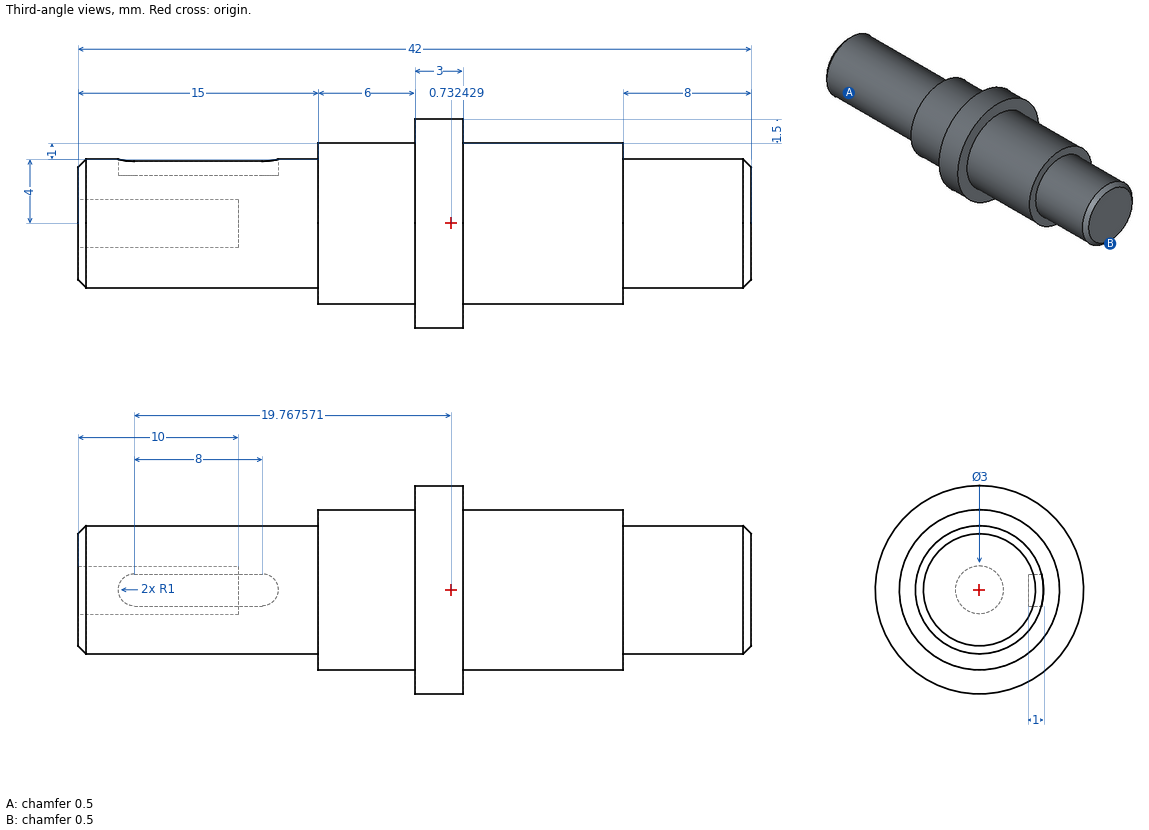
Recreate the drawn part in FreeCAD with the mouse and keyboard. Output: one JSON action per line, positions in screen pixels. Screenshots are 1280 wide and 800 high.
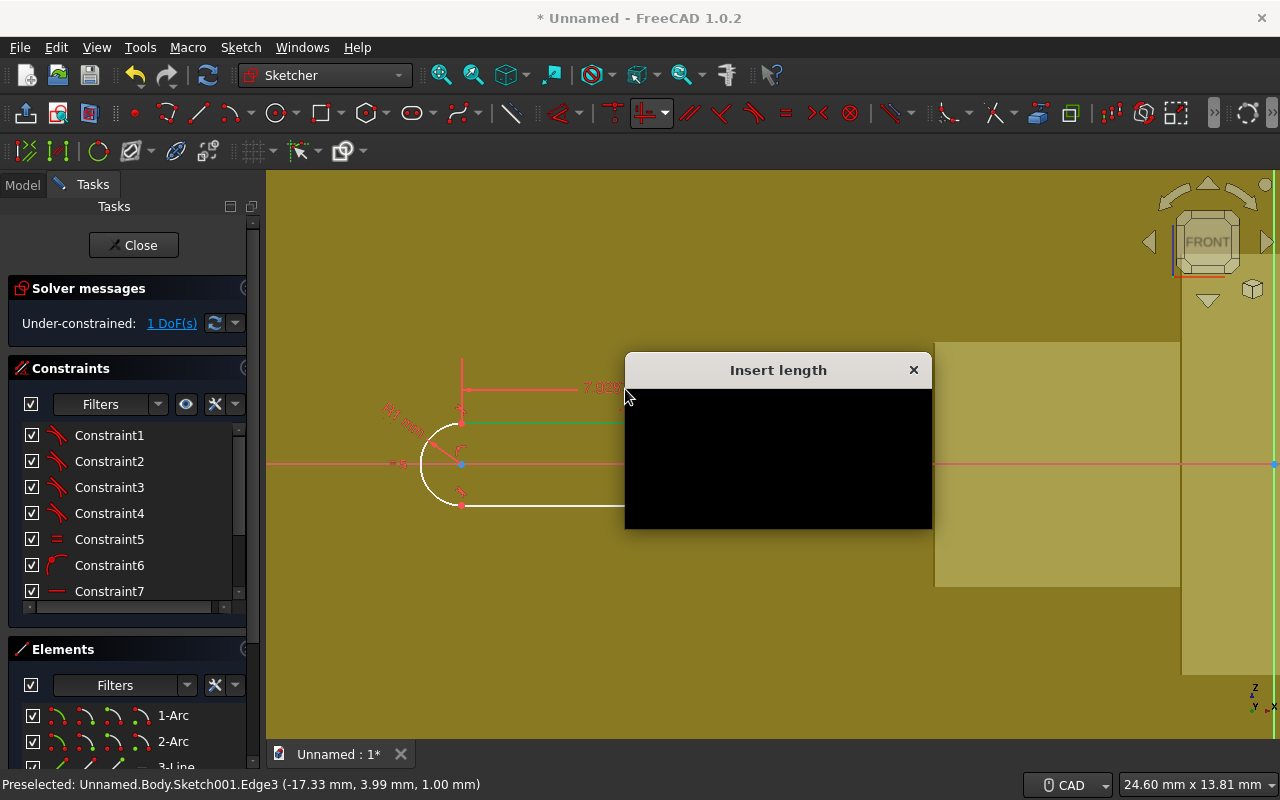
{"action": "type", "text": "8"}
{"action": "key", "text": "Return"}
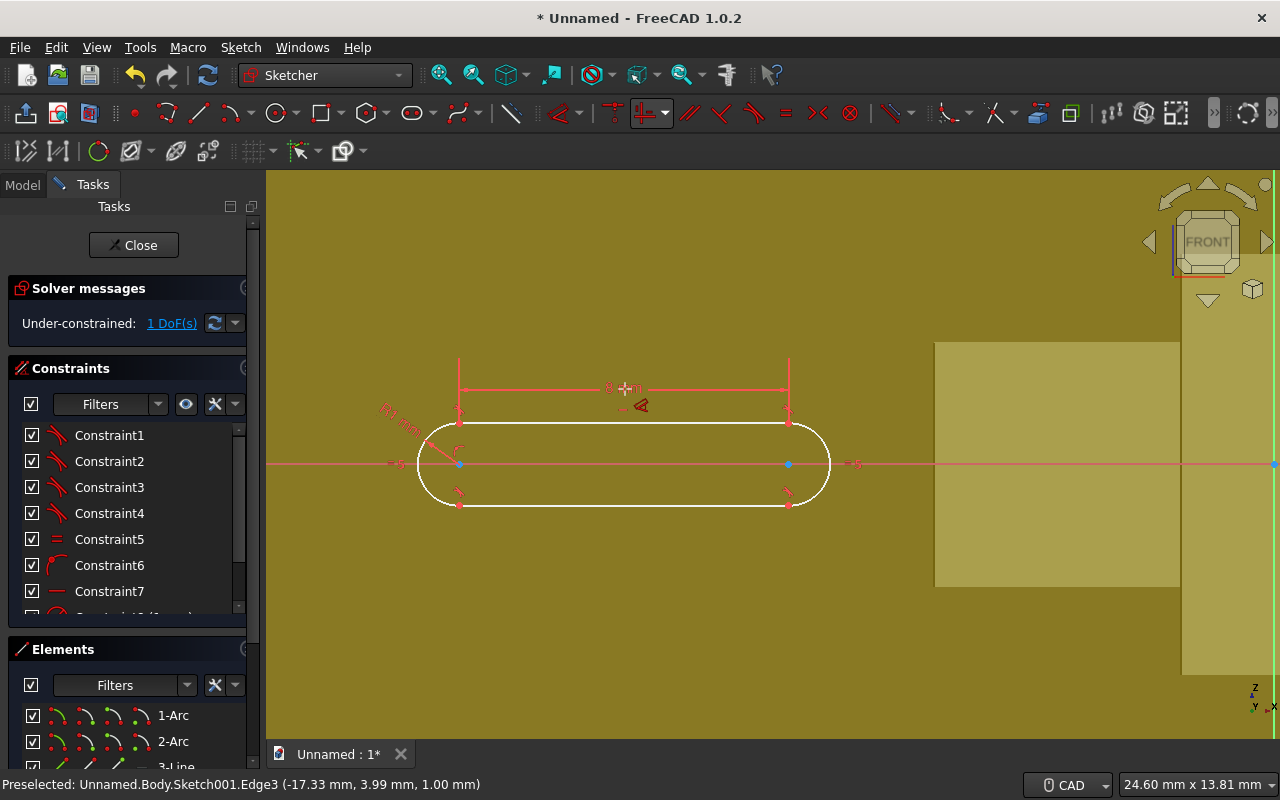
{"action": "left_click", "coordinate": [459, 423]}
{"action": "left_click", "coordinate": [787, 389]}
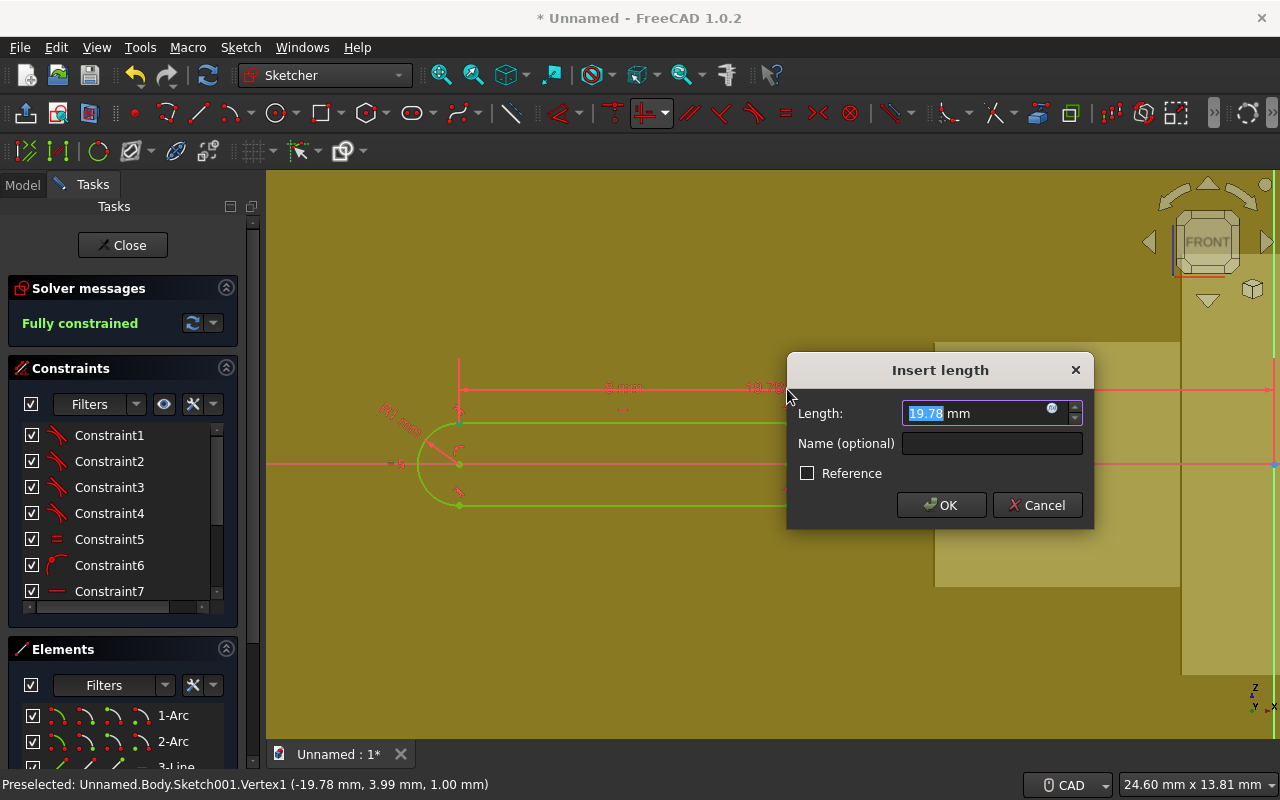
{"action": "type", "text": "19.767571"}
{"action": "key", "text": "Return"}
{"action": "key", "text": "Escape"}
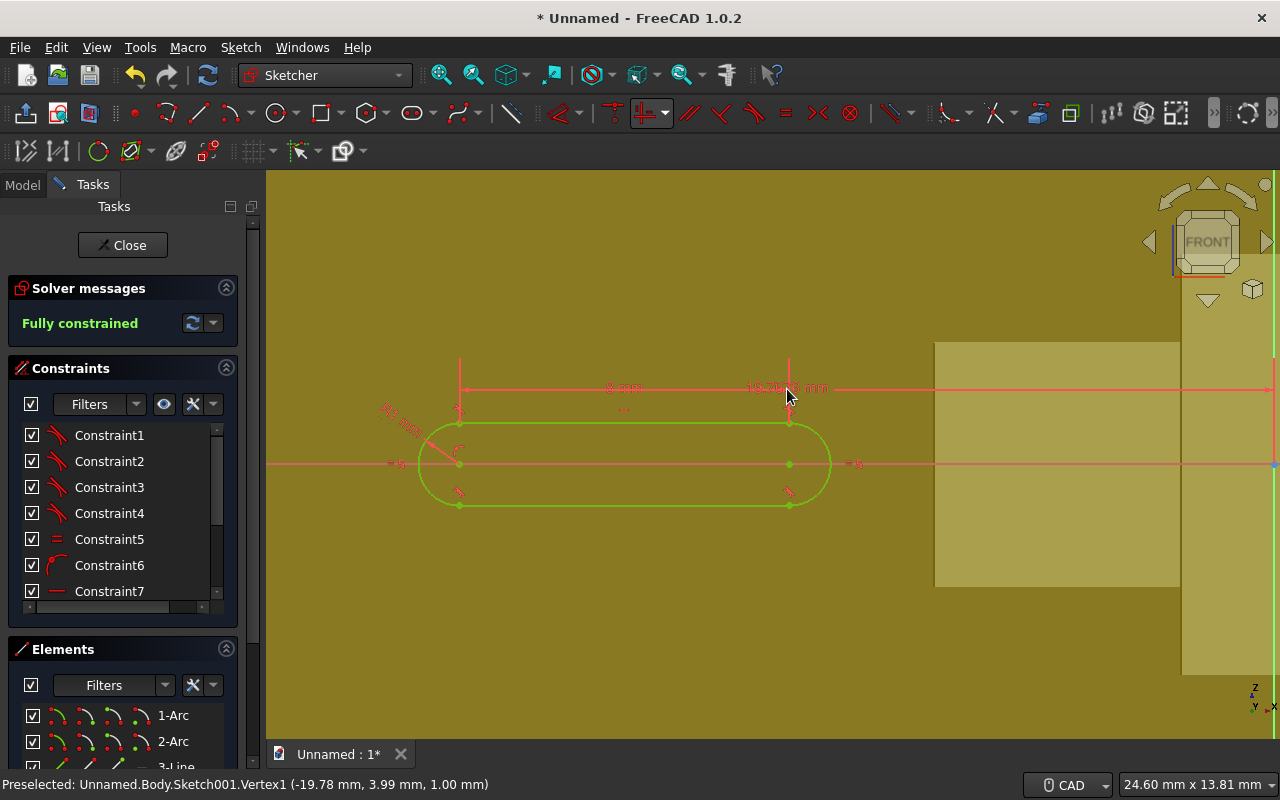
{"action": "left_click", "coordinate": [123, 245]}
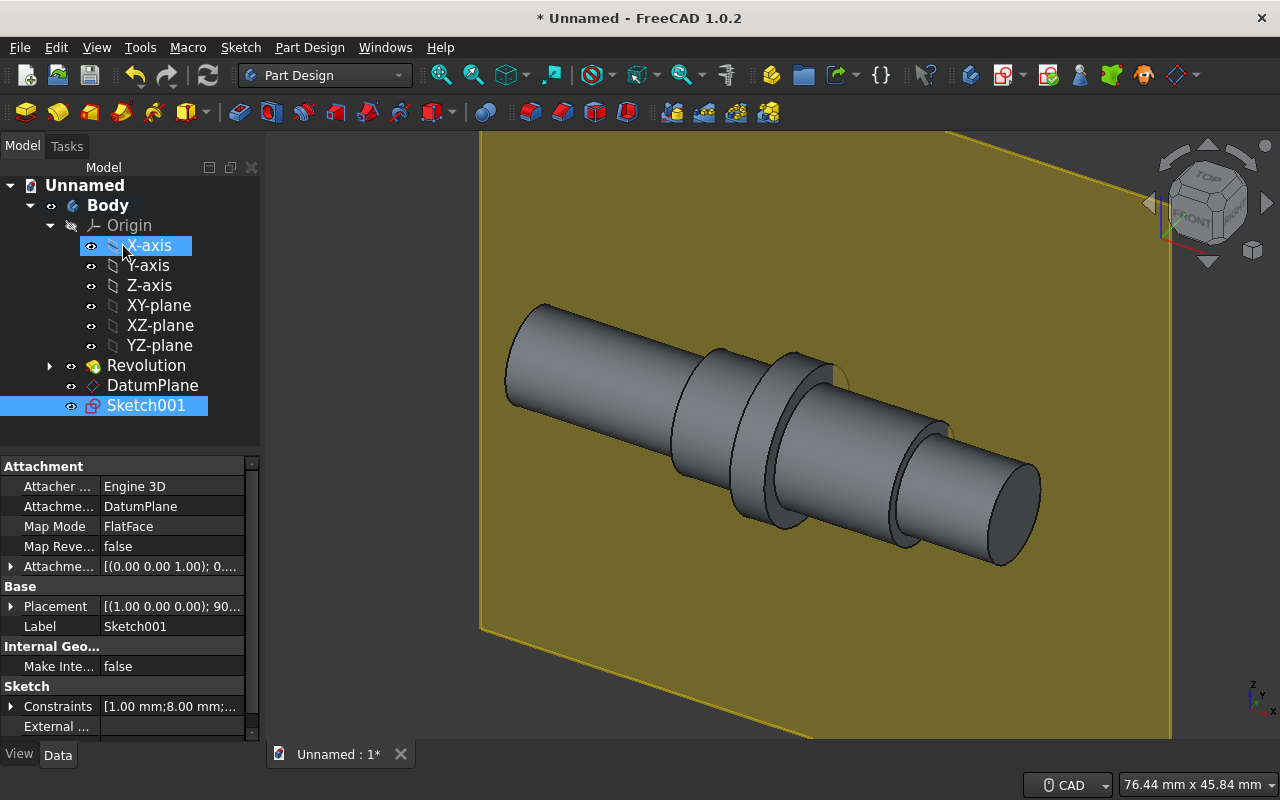
{"action": "left_click", "coordinate": [240, 112]}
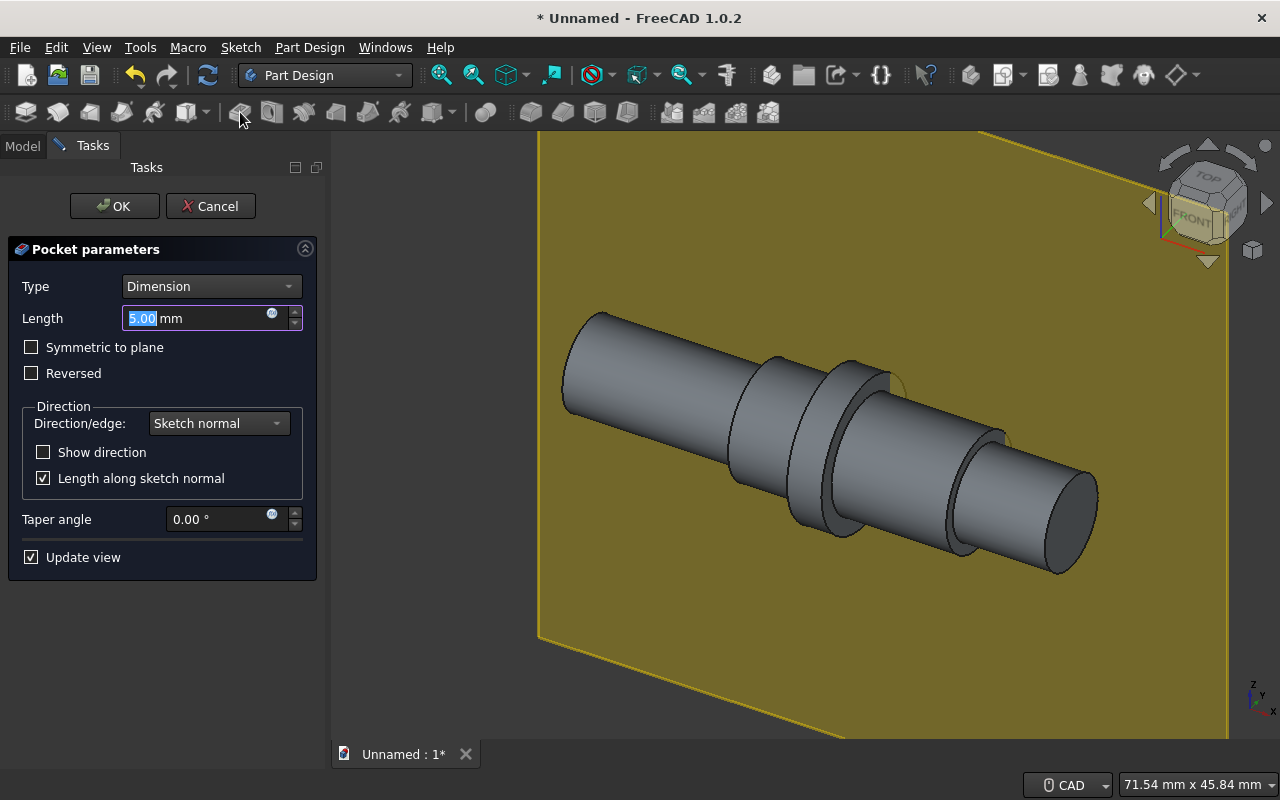
{"action": "type", "text": "1"}
{"action": "key", "text": "Tab"}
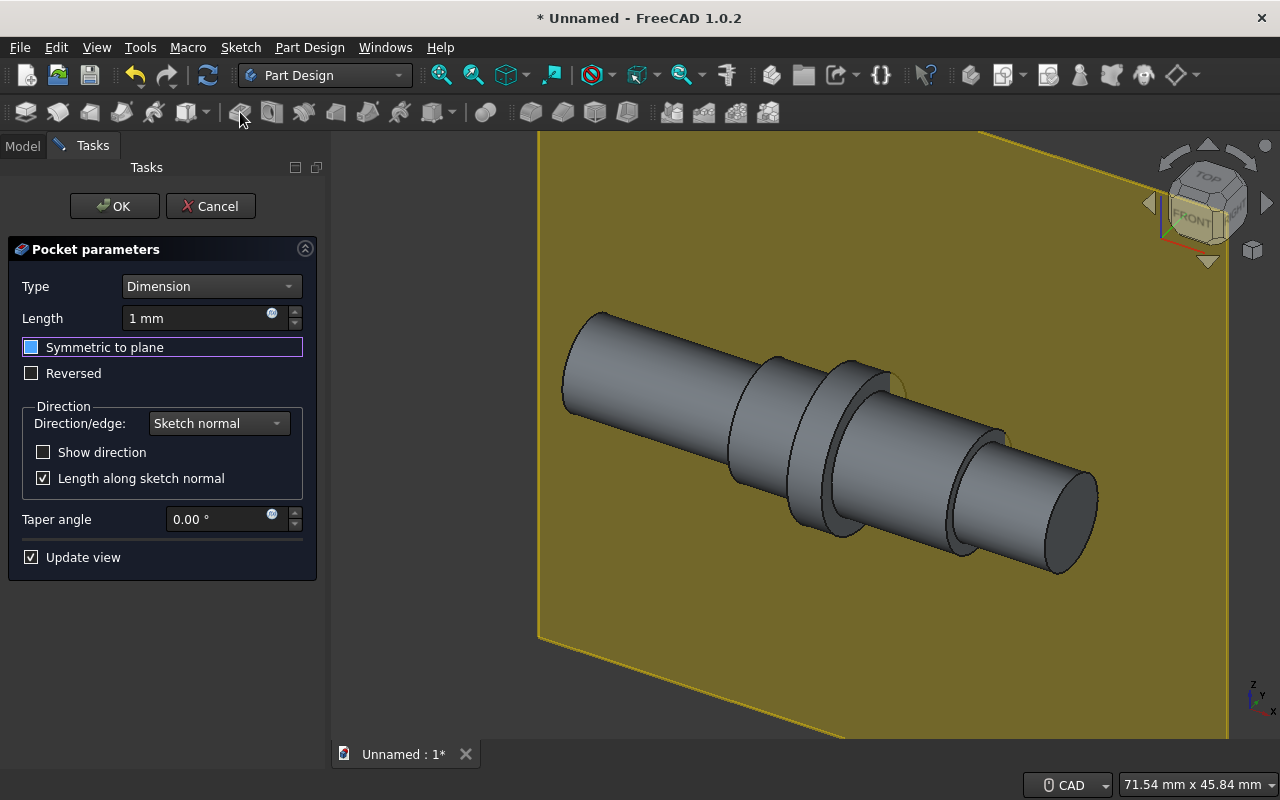
{"action": "left_click", "coordinate": [30, 373]}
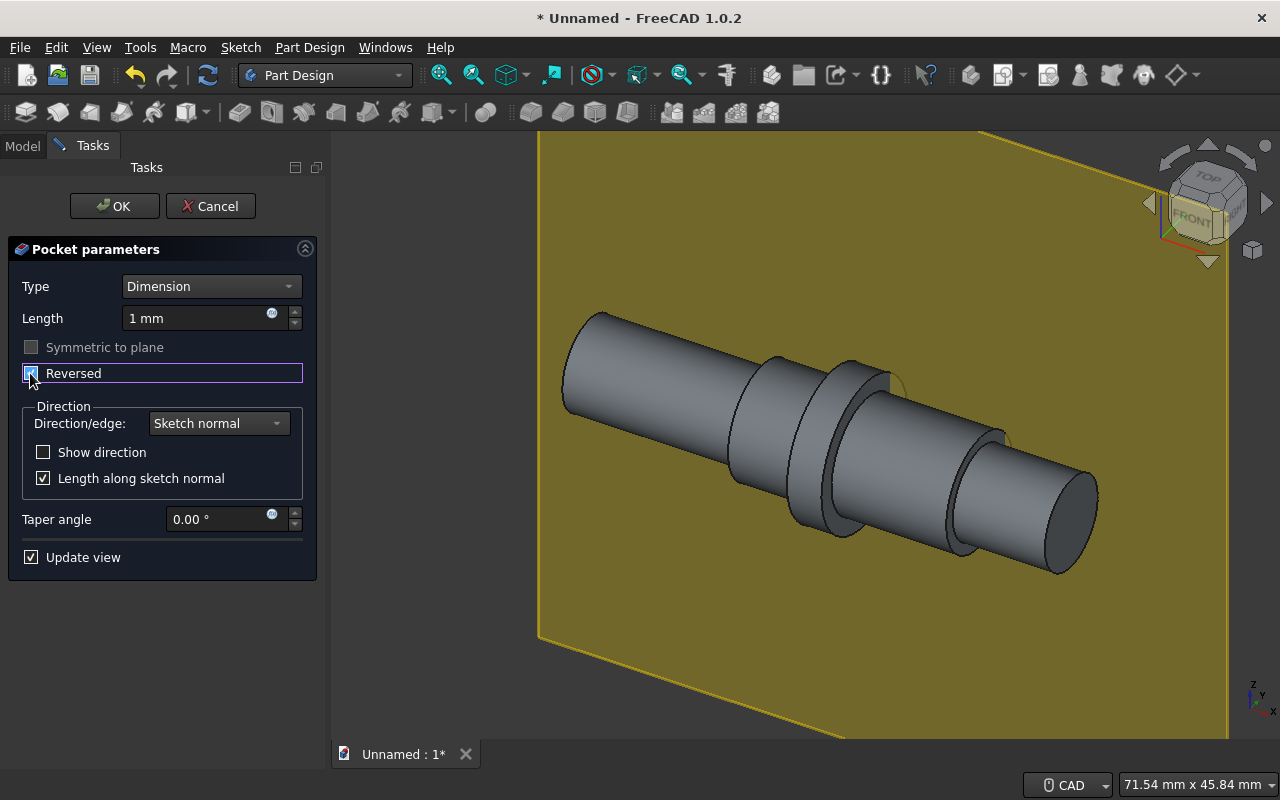
{"action": "left_click", "coordinate": [115, 206]}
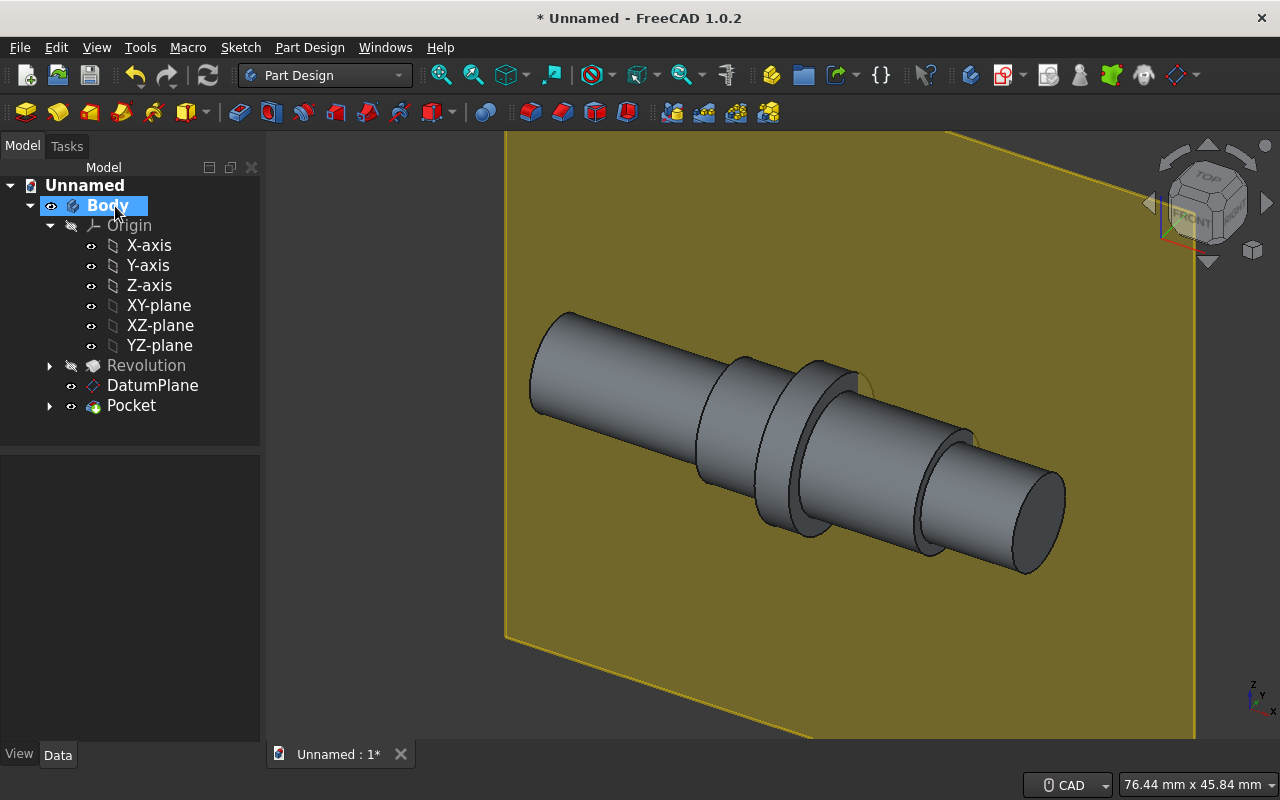
{"action": "left_click", "coordinate": [116, 386]}
{"action": "key", "text": "space"}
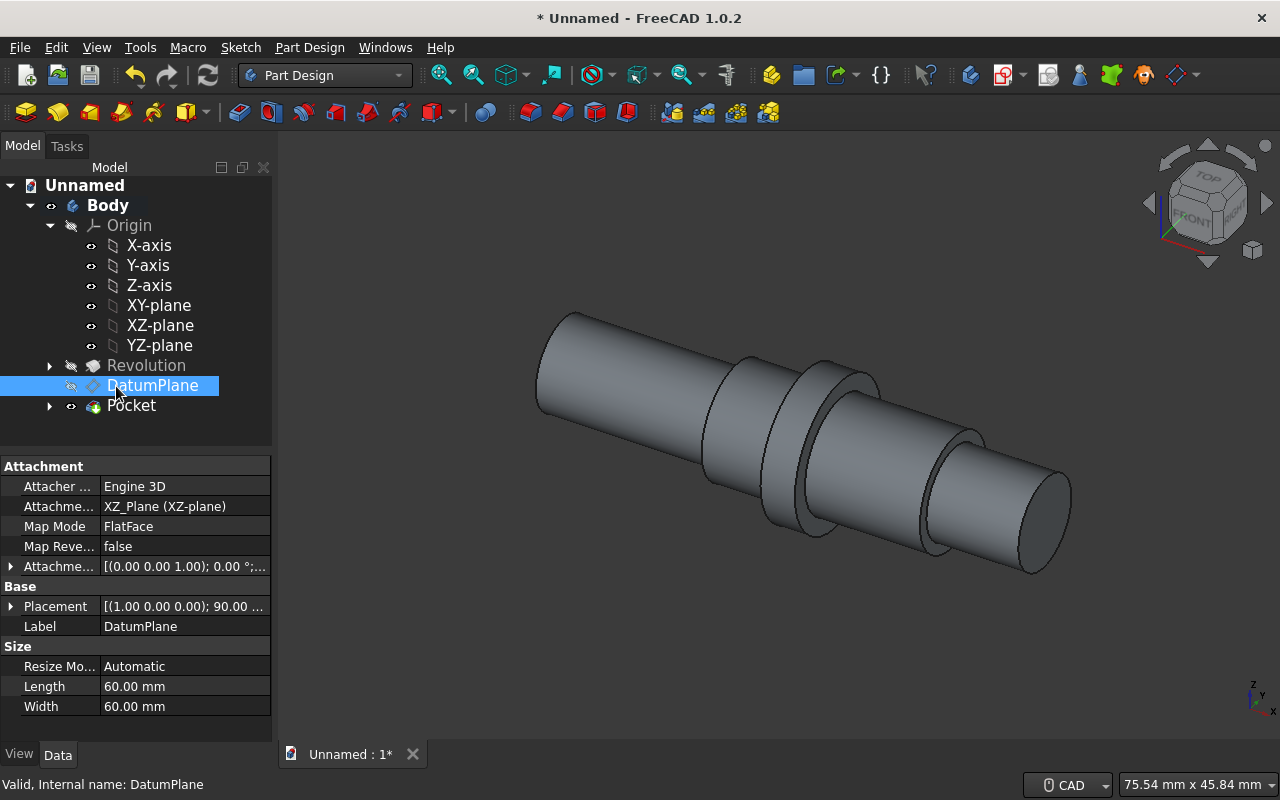
{"action": "key", "text": "6"}